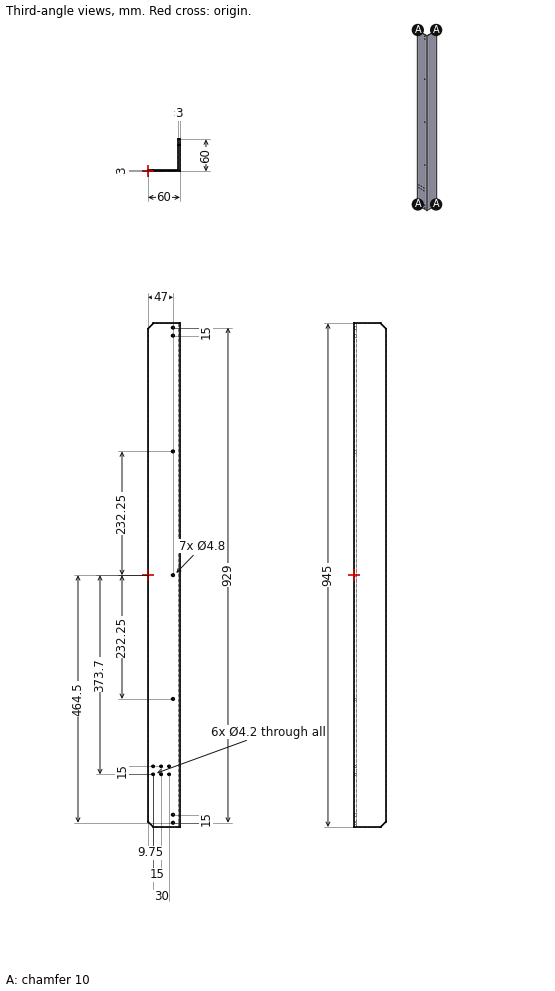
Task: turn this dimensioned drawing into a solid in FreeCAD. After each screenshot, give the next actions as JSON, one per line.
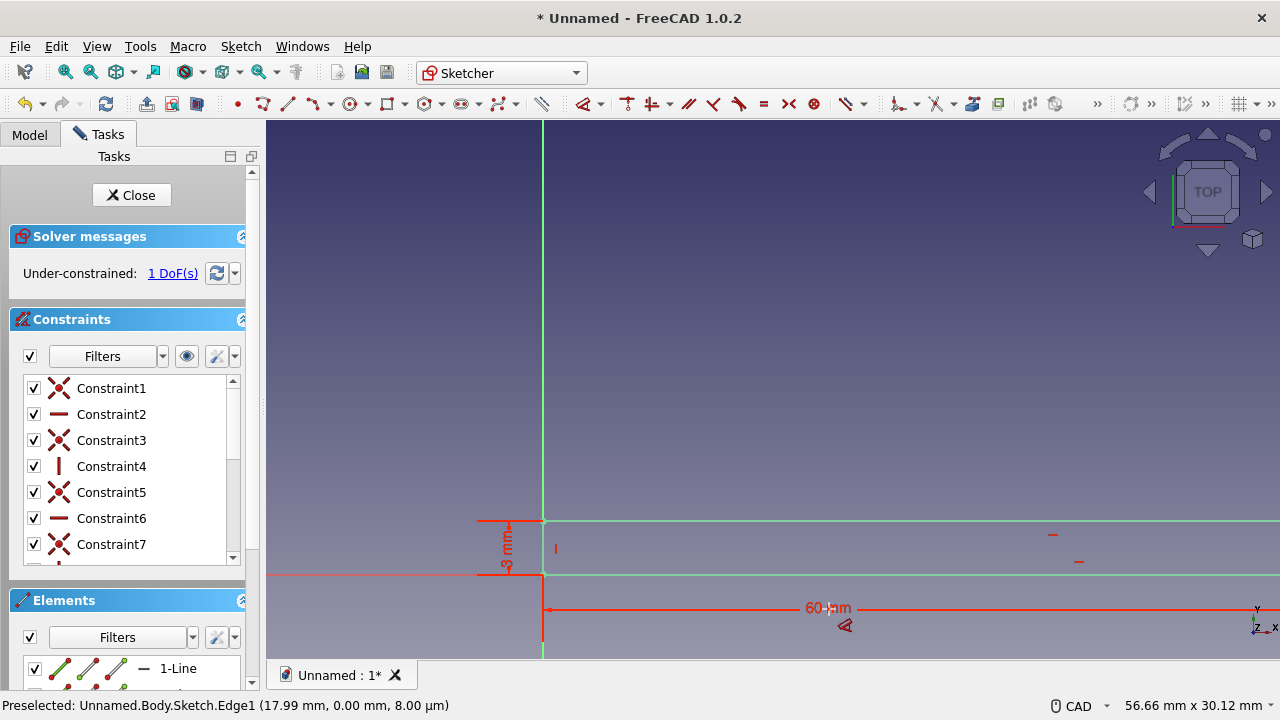
{"action": "scroll", "coordinate": [543, 541], "scroll_direction": "down", "scroll_amount": 6}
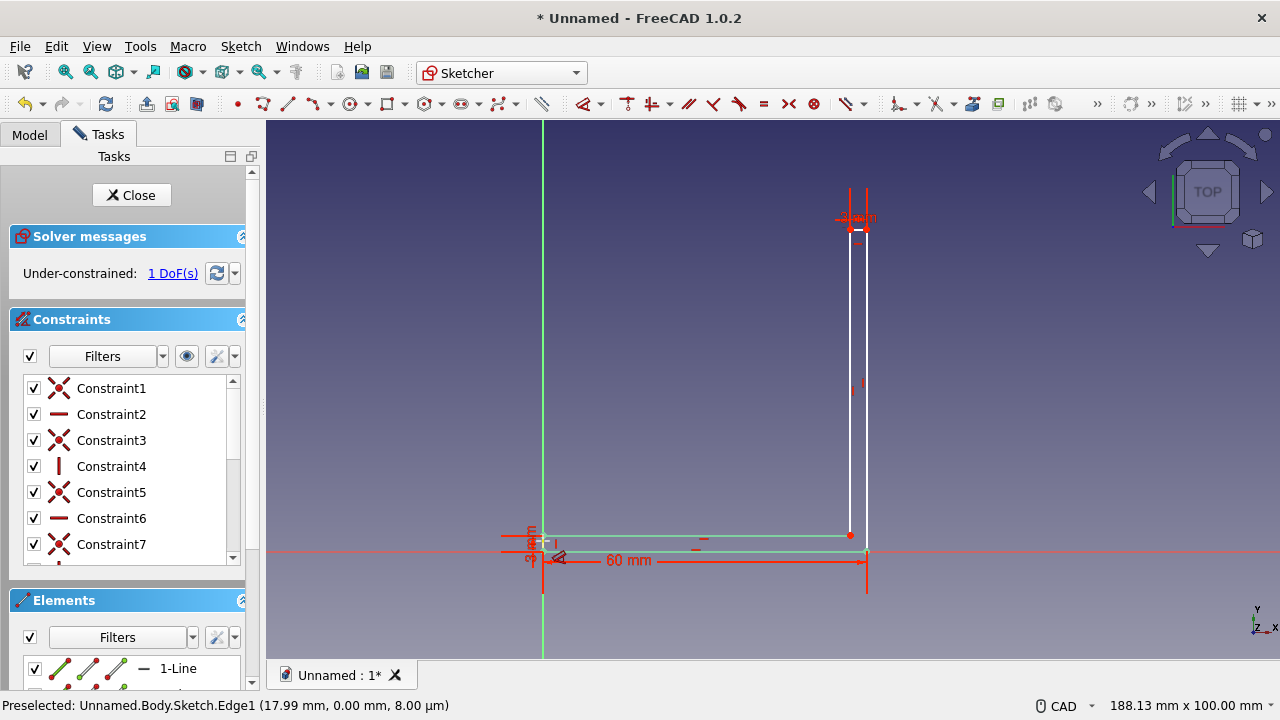
{"action": "left_click", "coordinate": [867, 455]}
{"action": "left_click", "coordinate": [901, 391]}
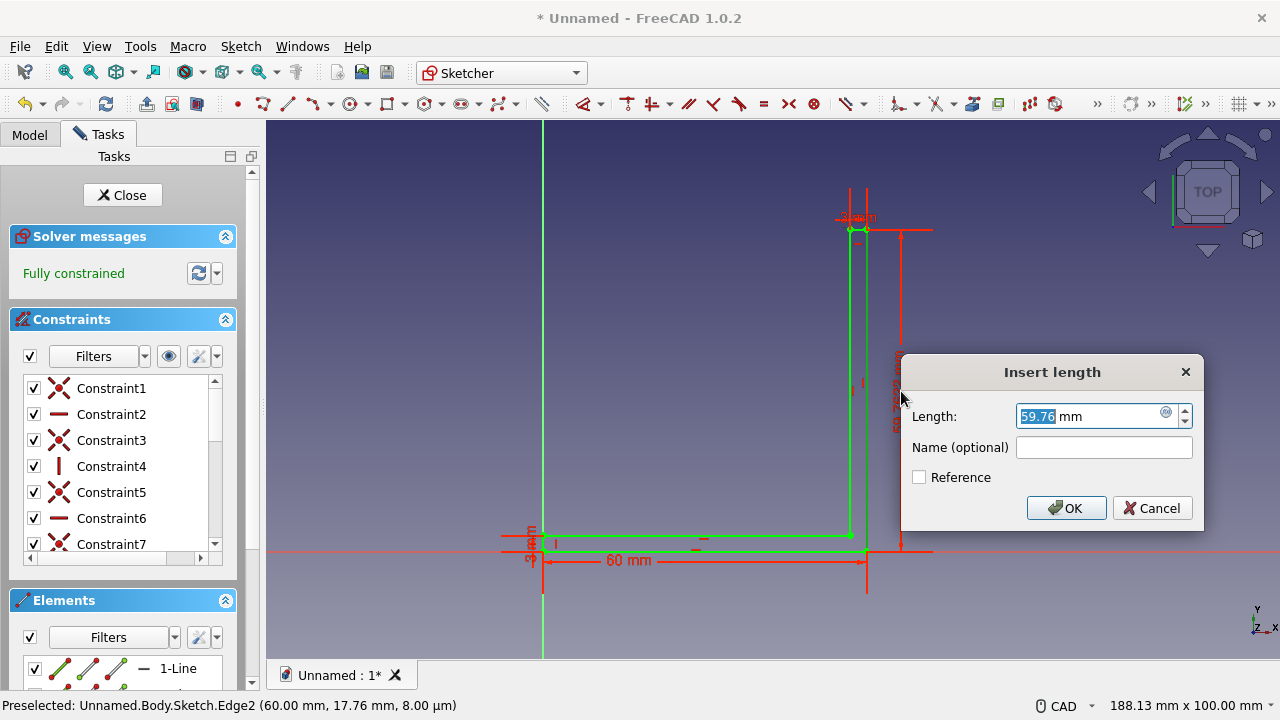
{"action": "type", "text": "60"}
{"action": "key", "text": "Return"}
{"action": "key", "text": "Escape"}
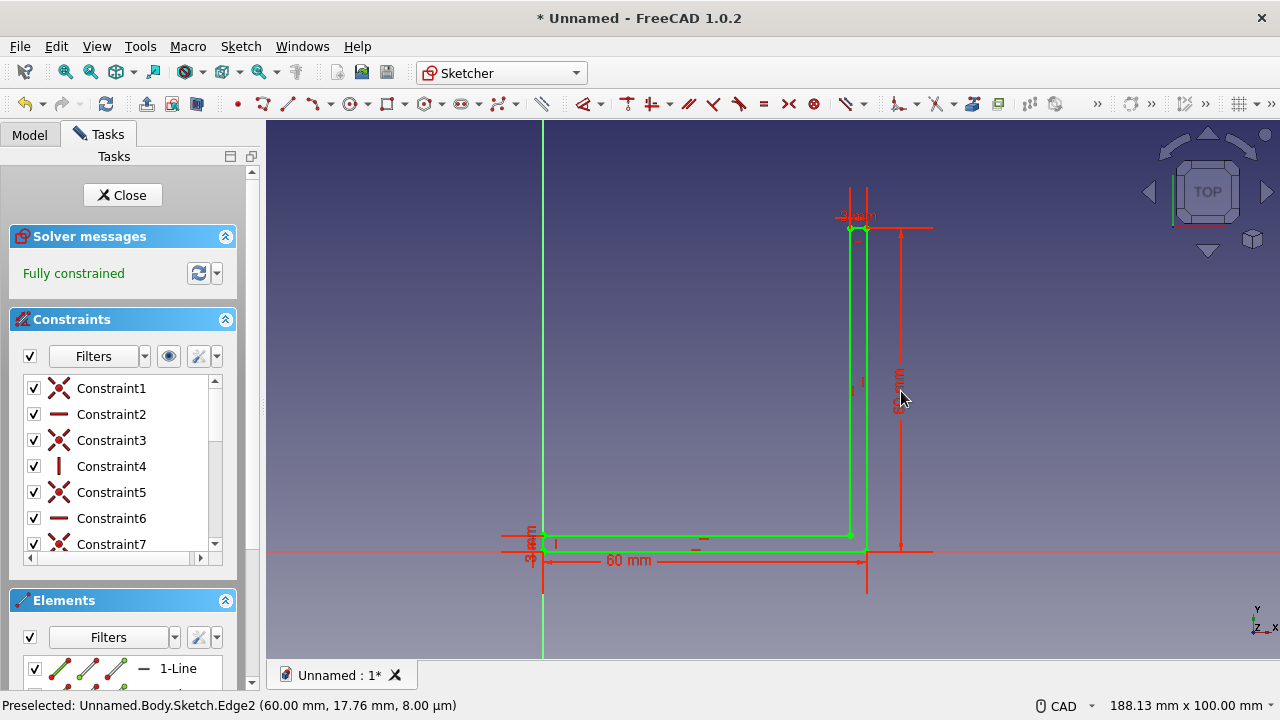
{"action": "left_click", "coordinate": [123, 195]}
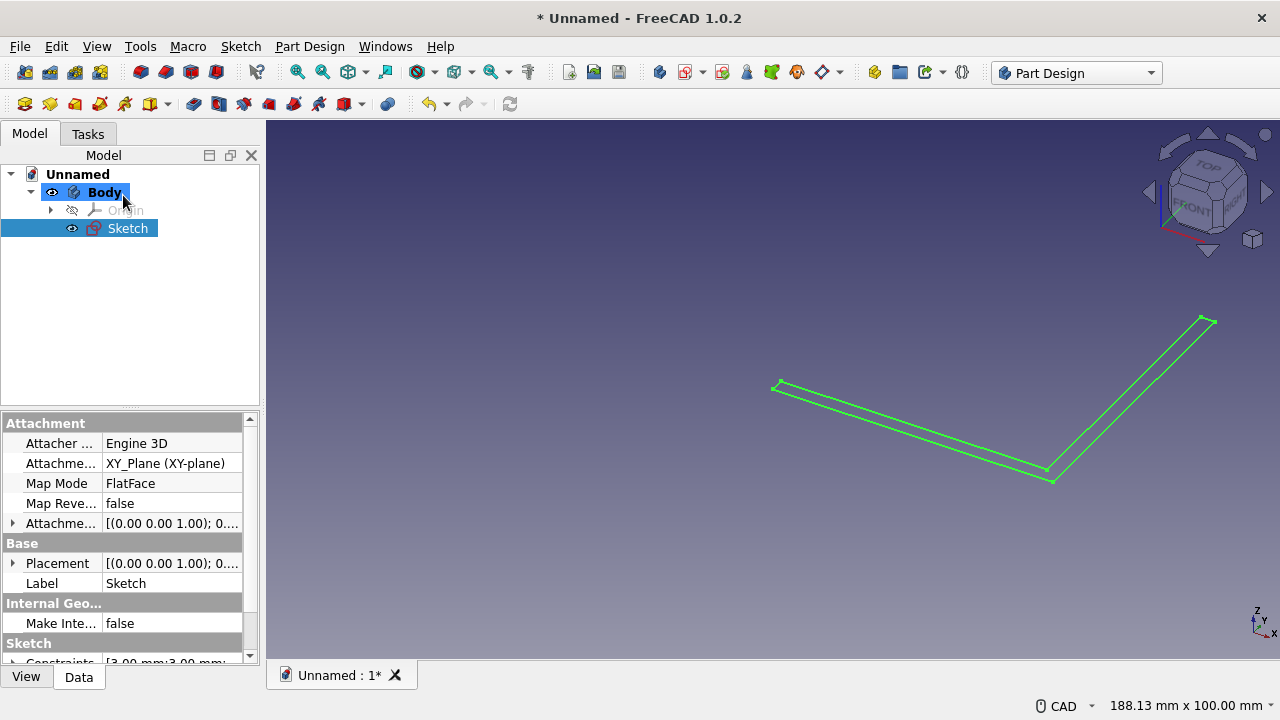
{"action": "left_click", "coordinate": [25, 104]}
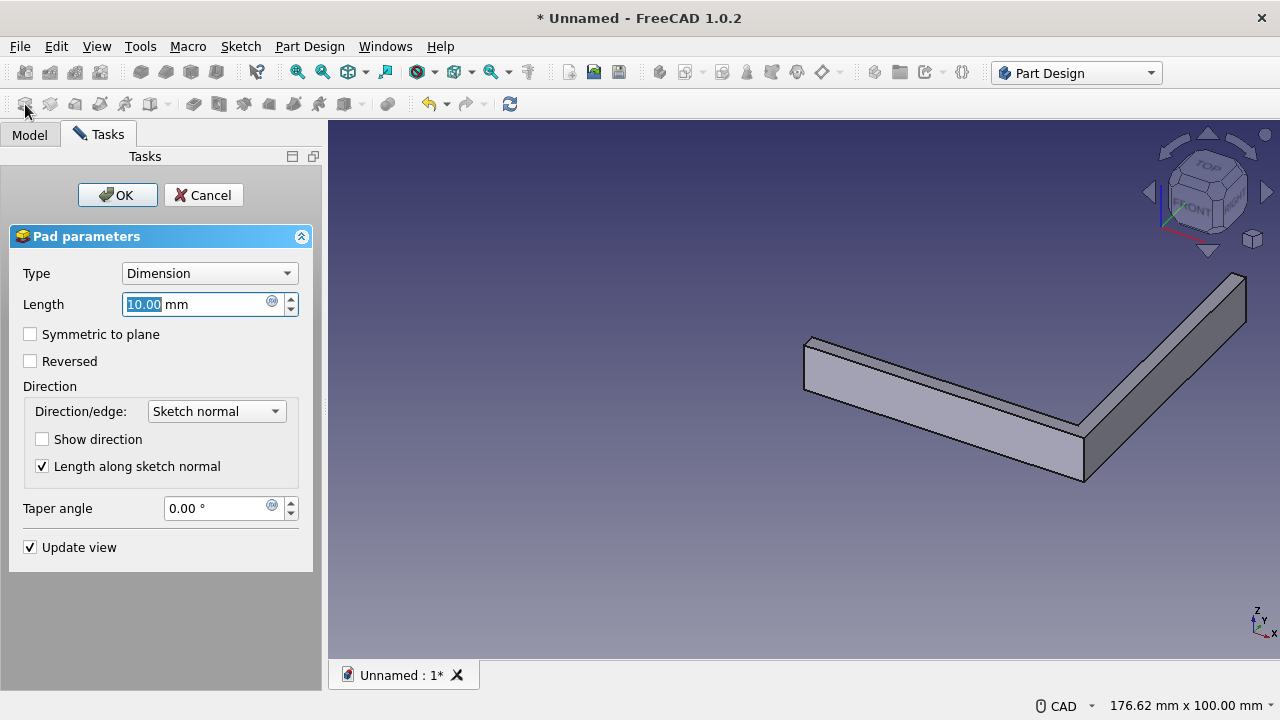
{"action": "type", "text": "945"}
{"action": "key", "text": "Tab"}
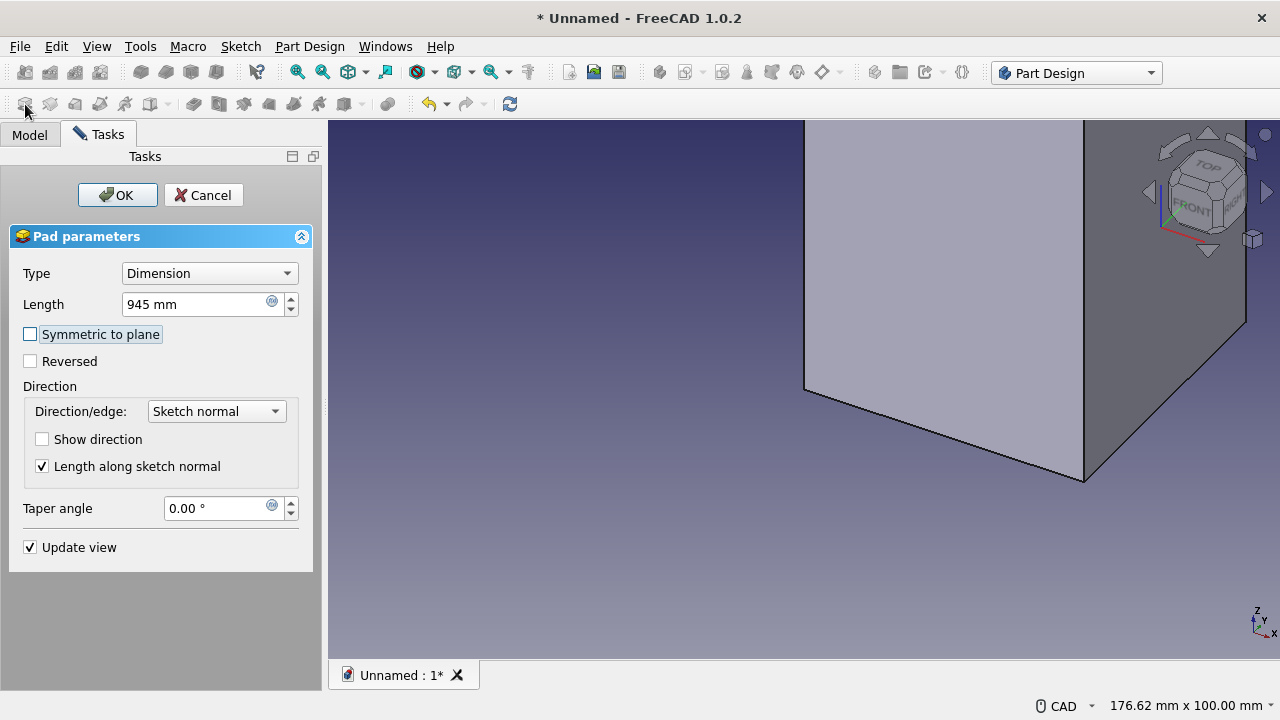
{"action": "left_click", "coordinate": [31, 334]}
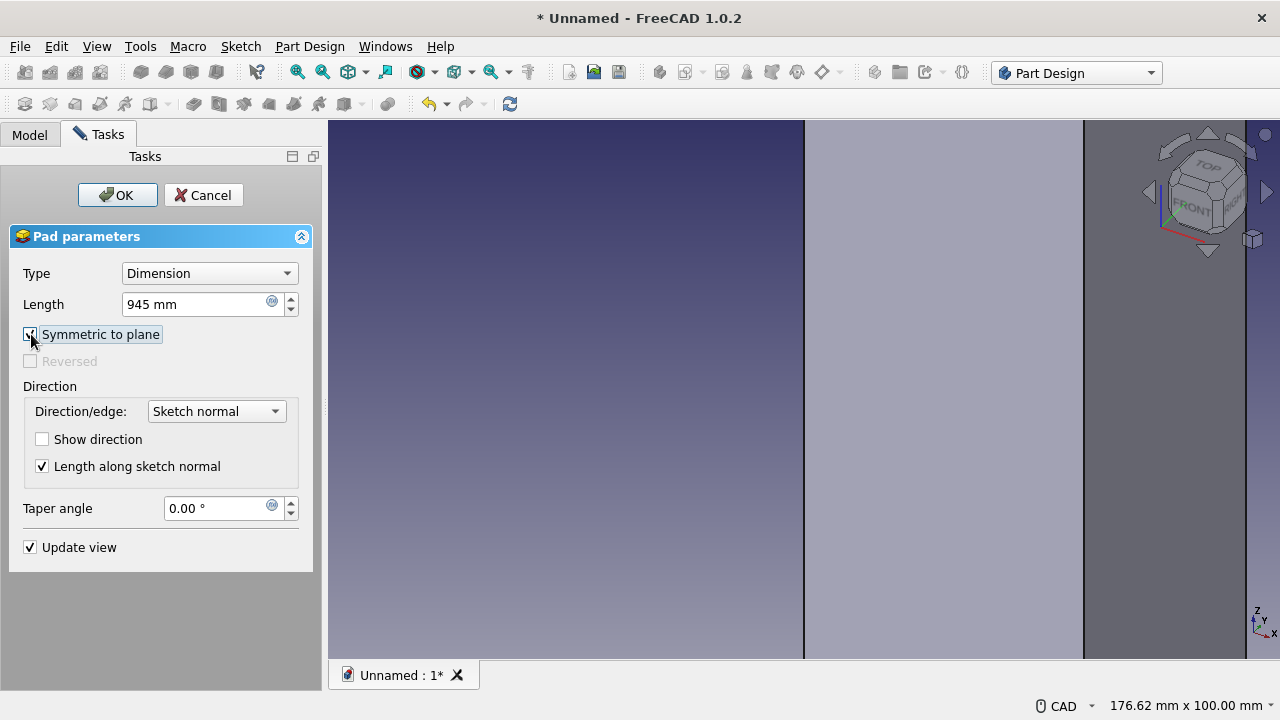
{"action": "left_click", "coordinate": [118, 195]}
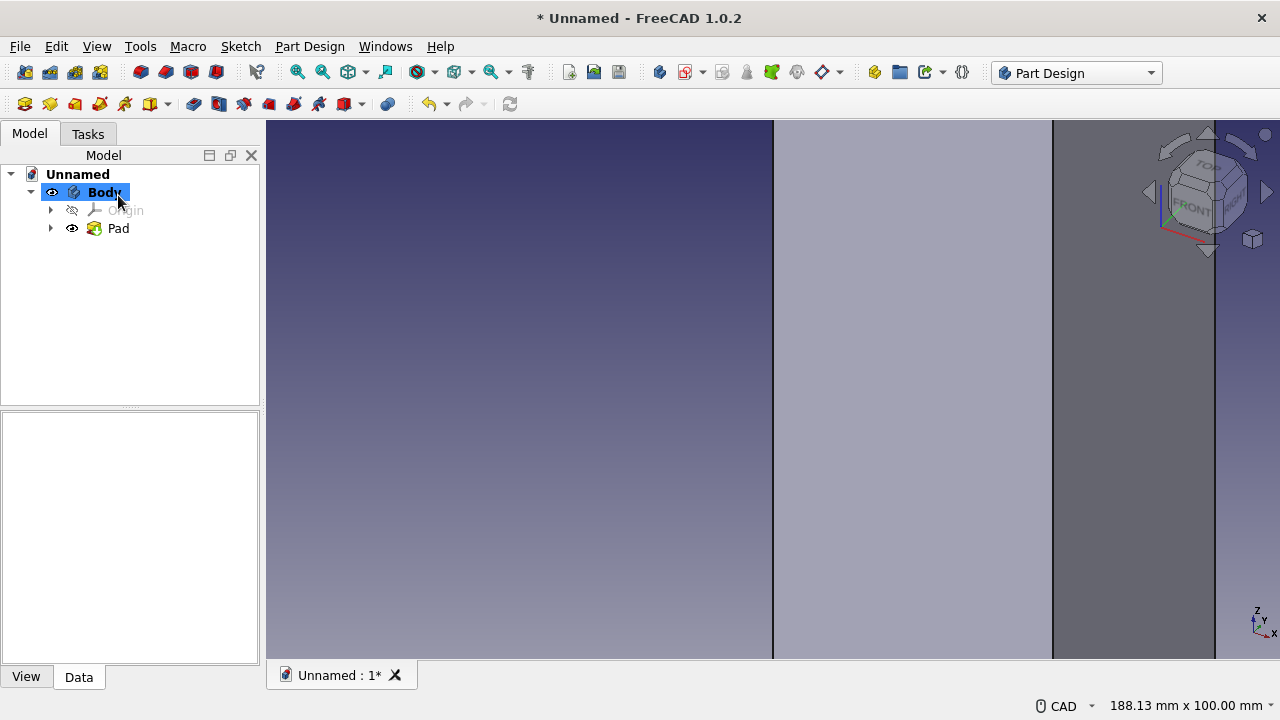
{"action": "left_click", "coordinate": [298, 72]}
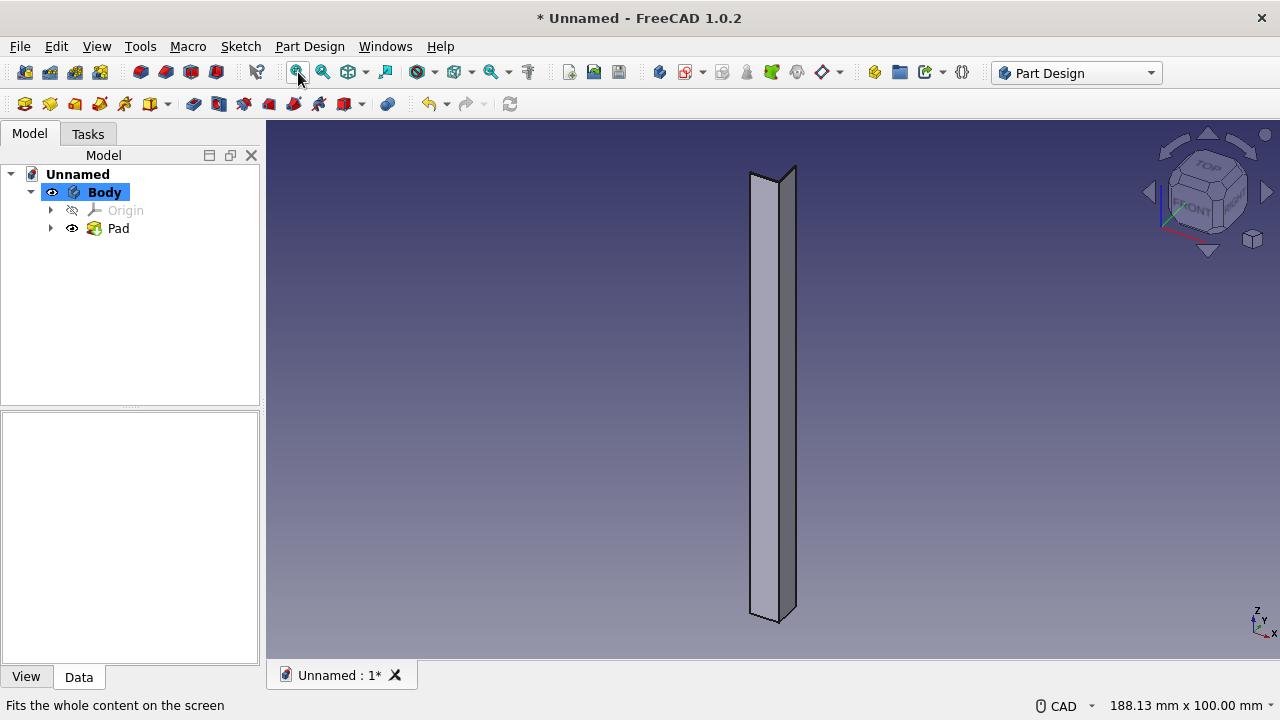
{"action": "key", "text": "4"}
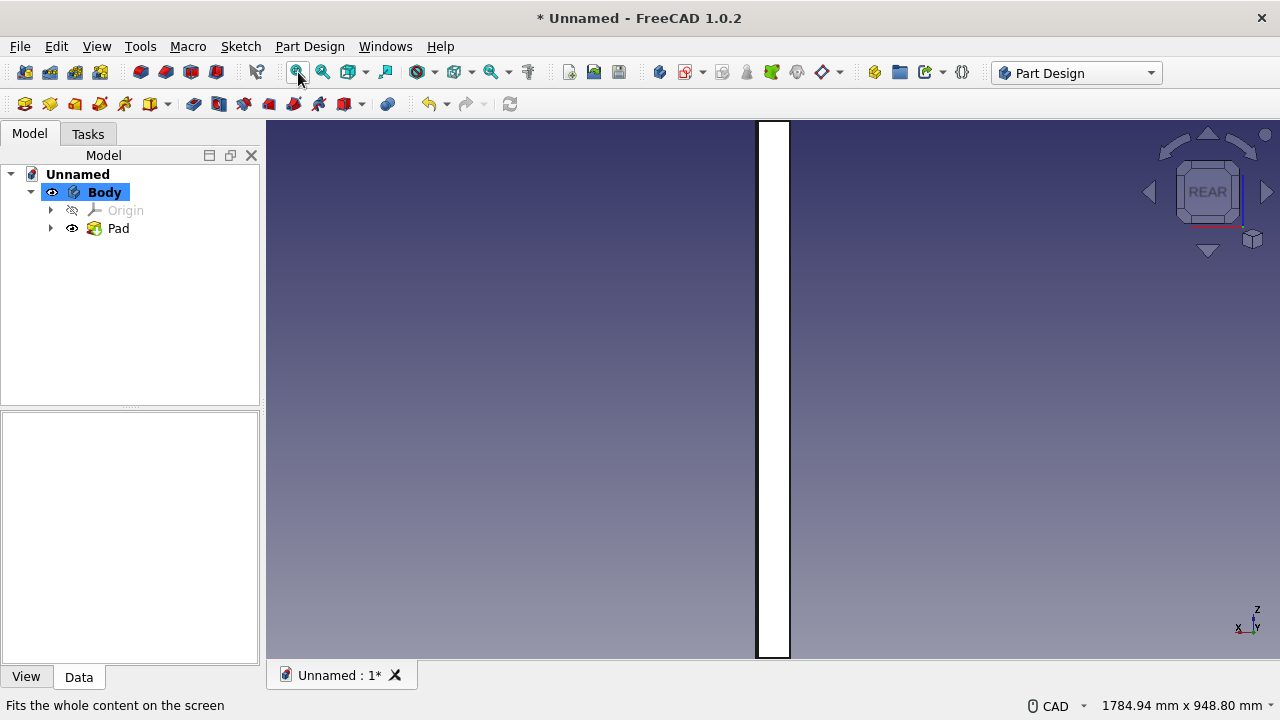
{"action": "left_click", "coordinate": [774, 158]}